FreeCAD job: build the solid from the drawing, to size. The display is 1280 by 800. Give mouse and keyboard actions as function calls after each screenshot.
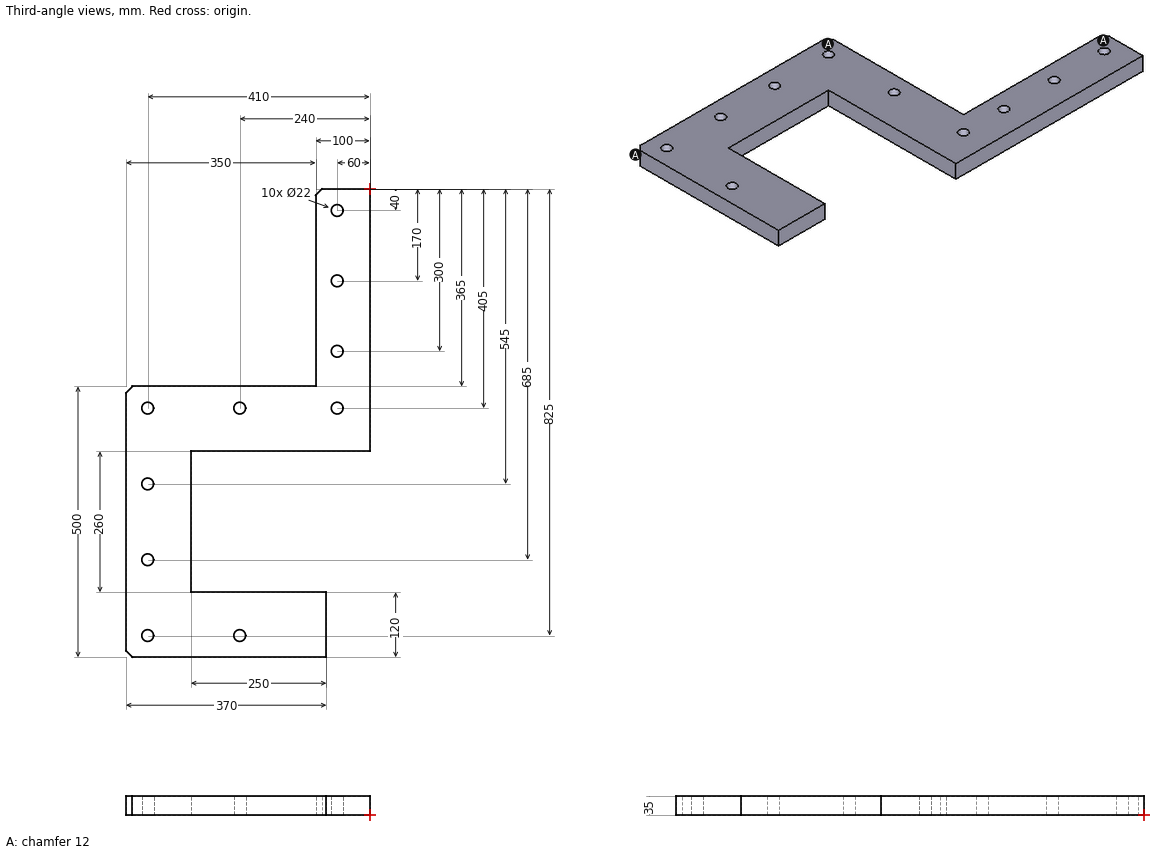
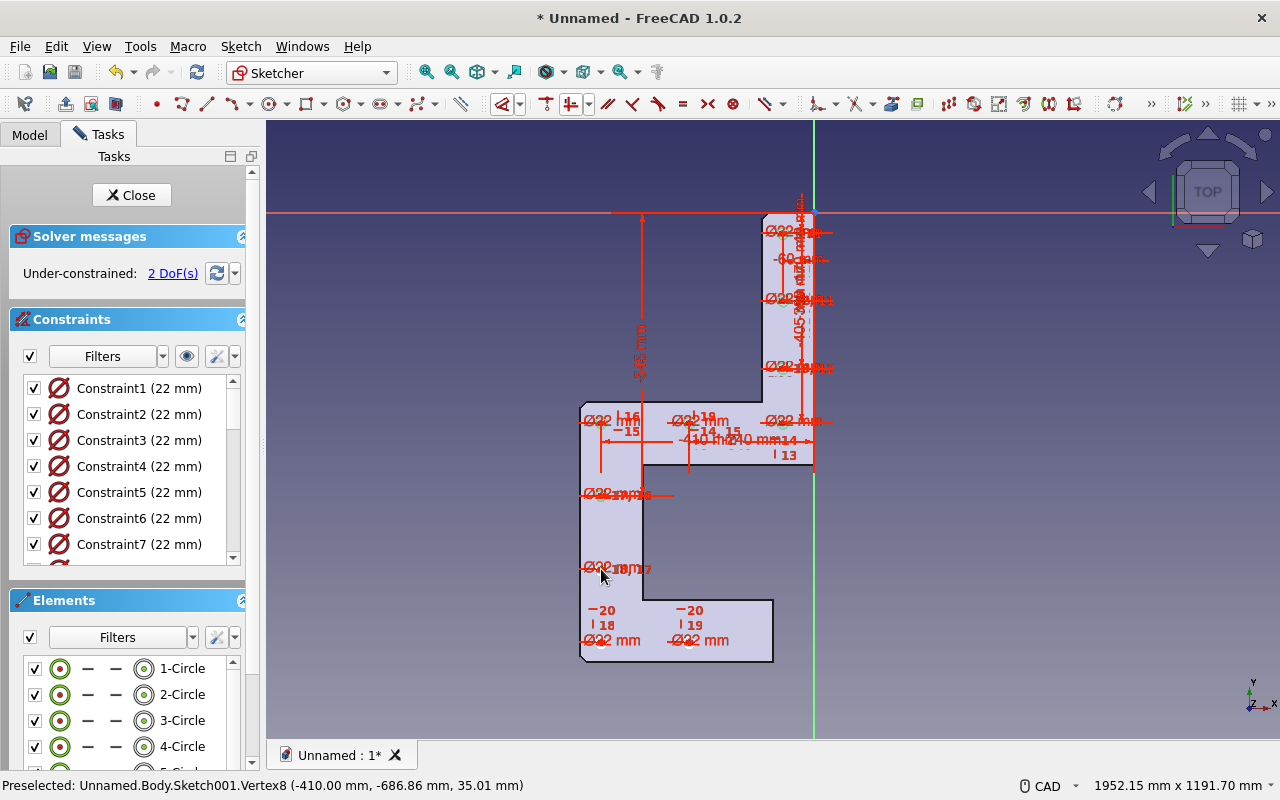
click(520, 104)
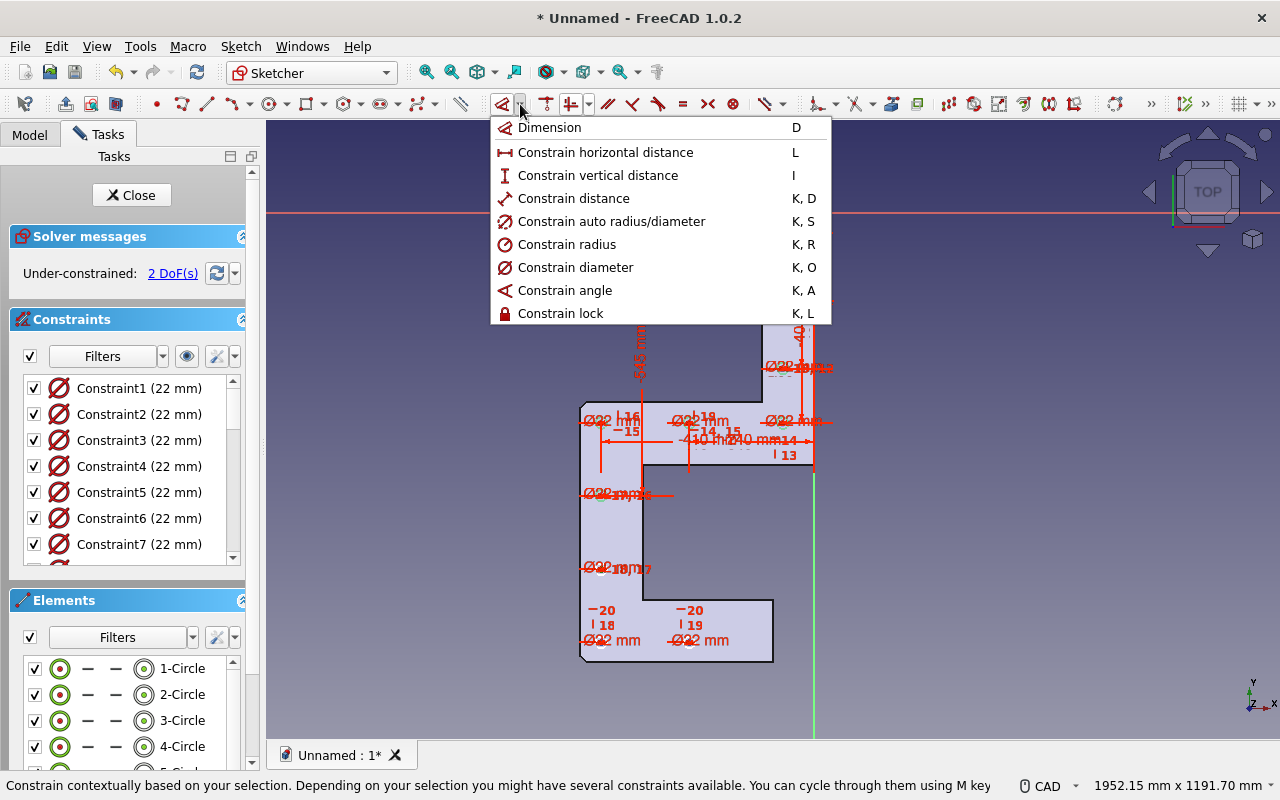
click(661, 176)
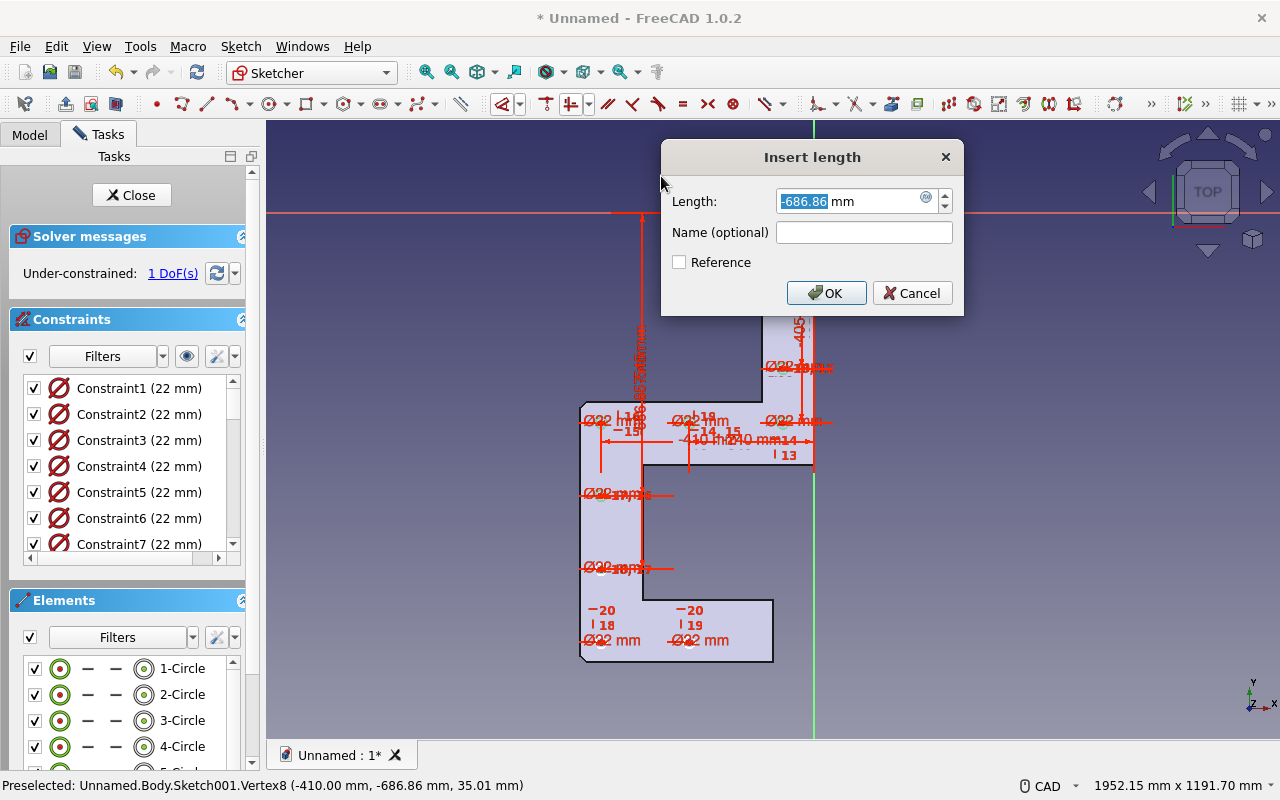
text(-685)
key(Return)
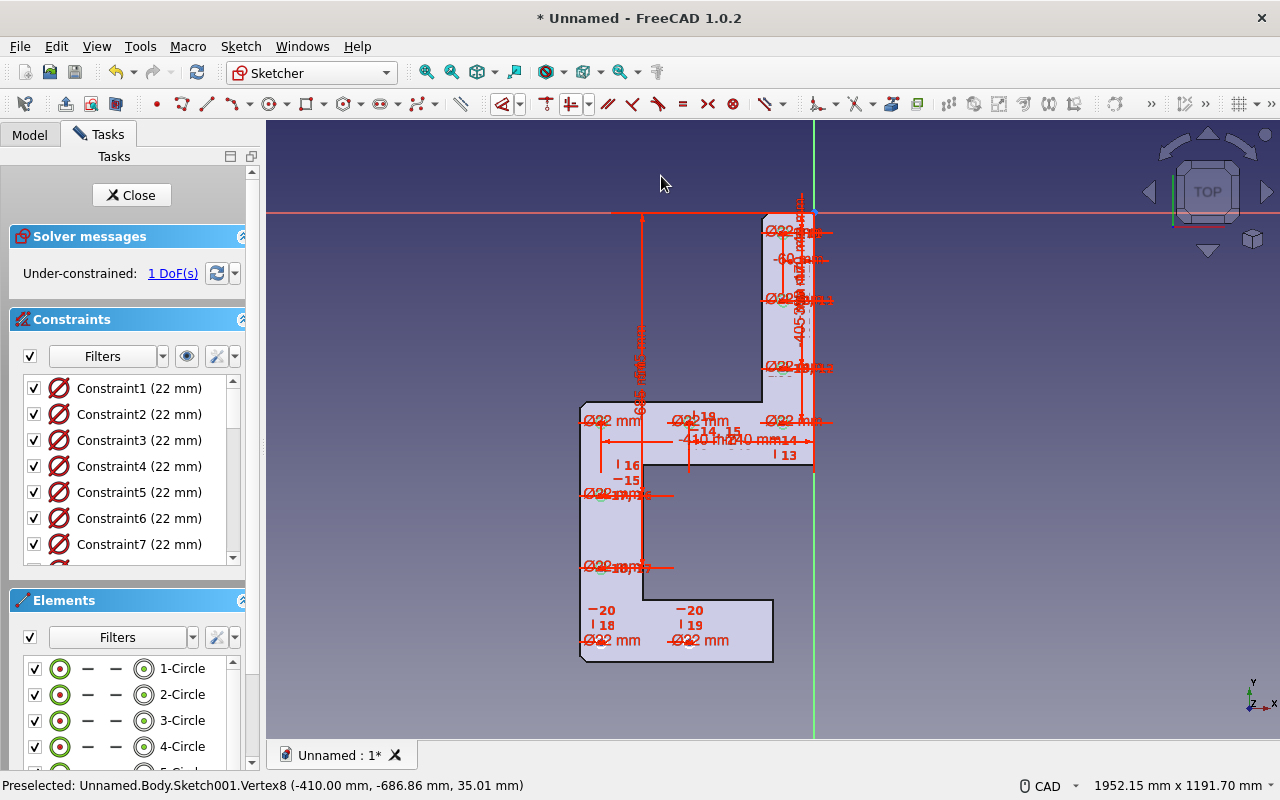
click(601, 642)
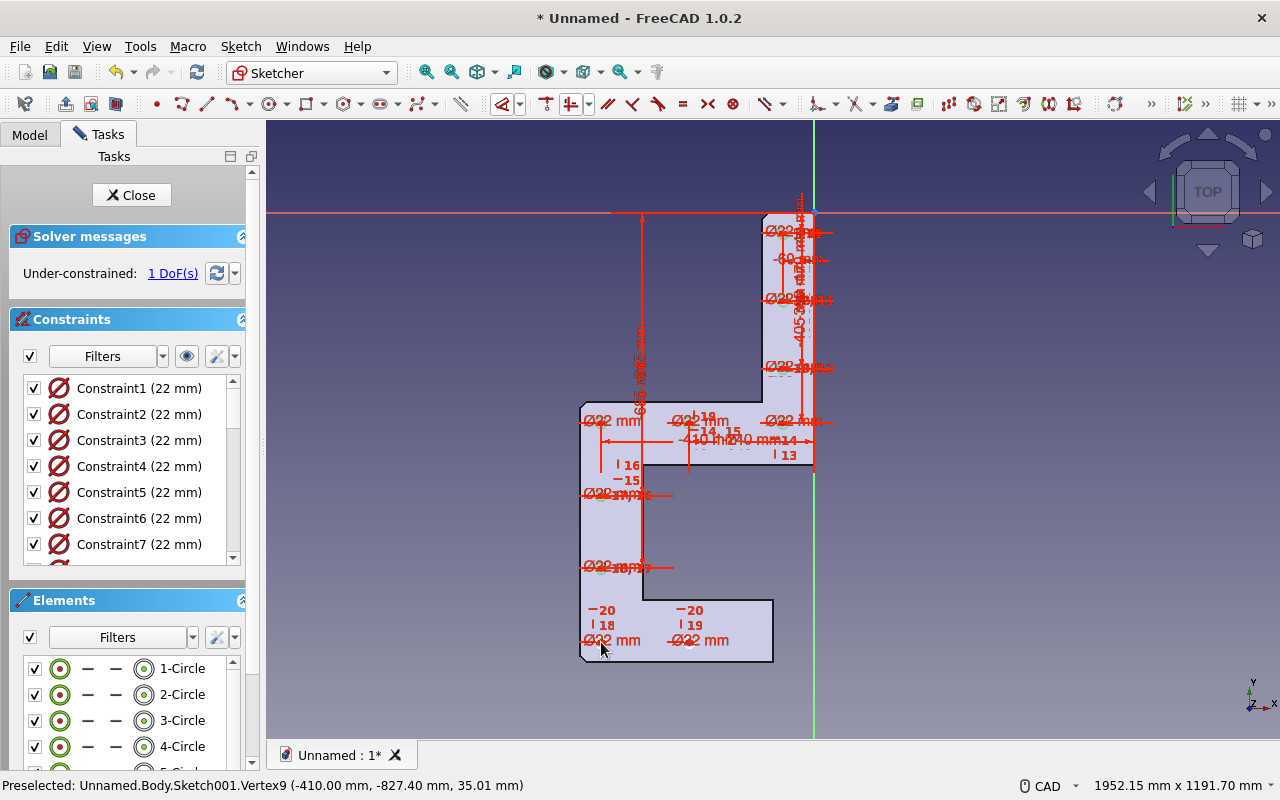
click(520, 104)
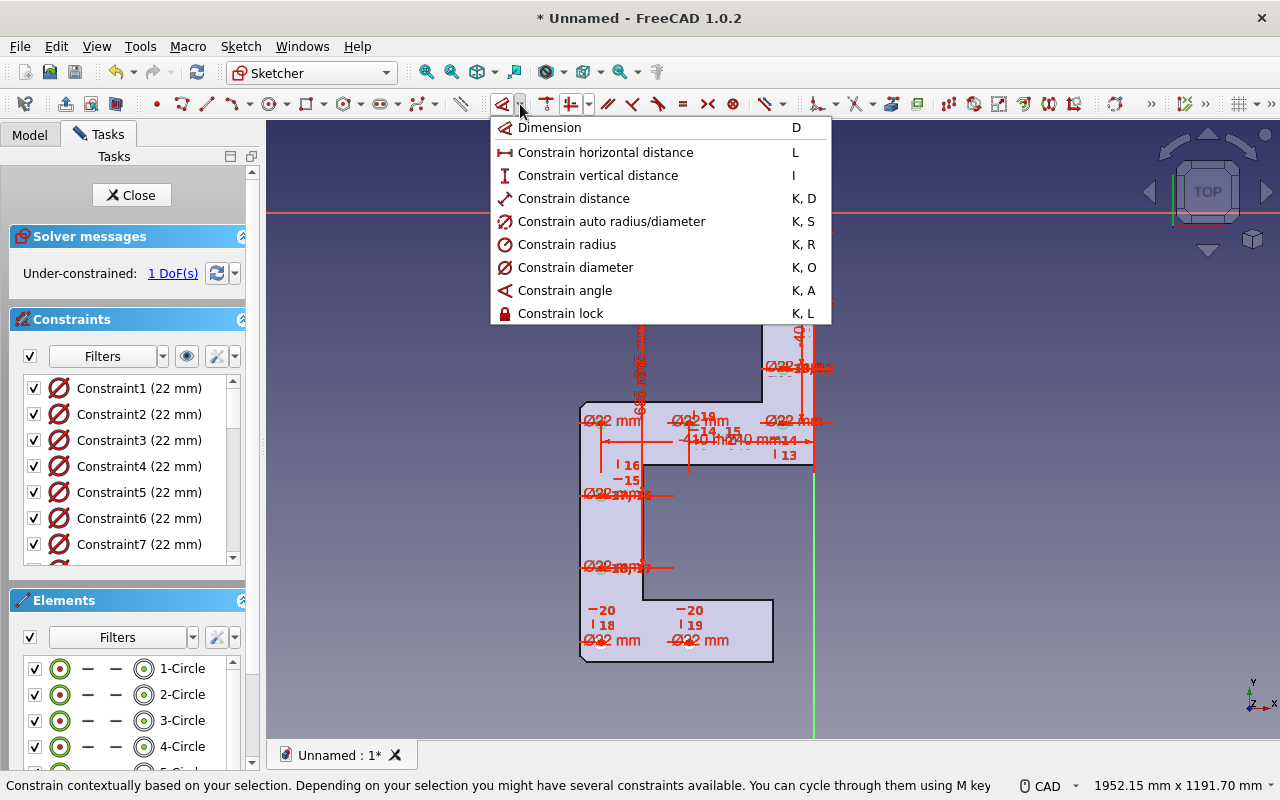
click(661, 176)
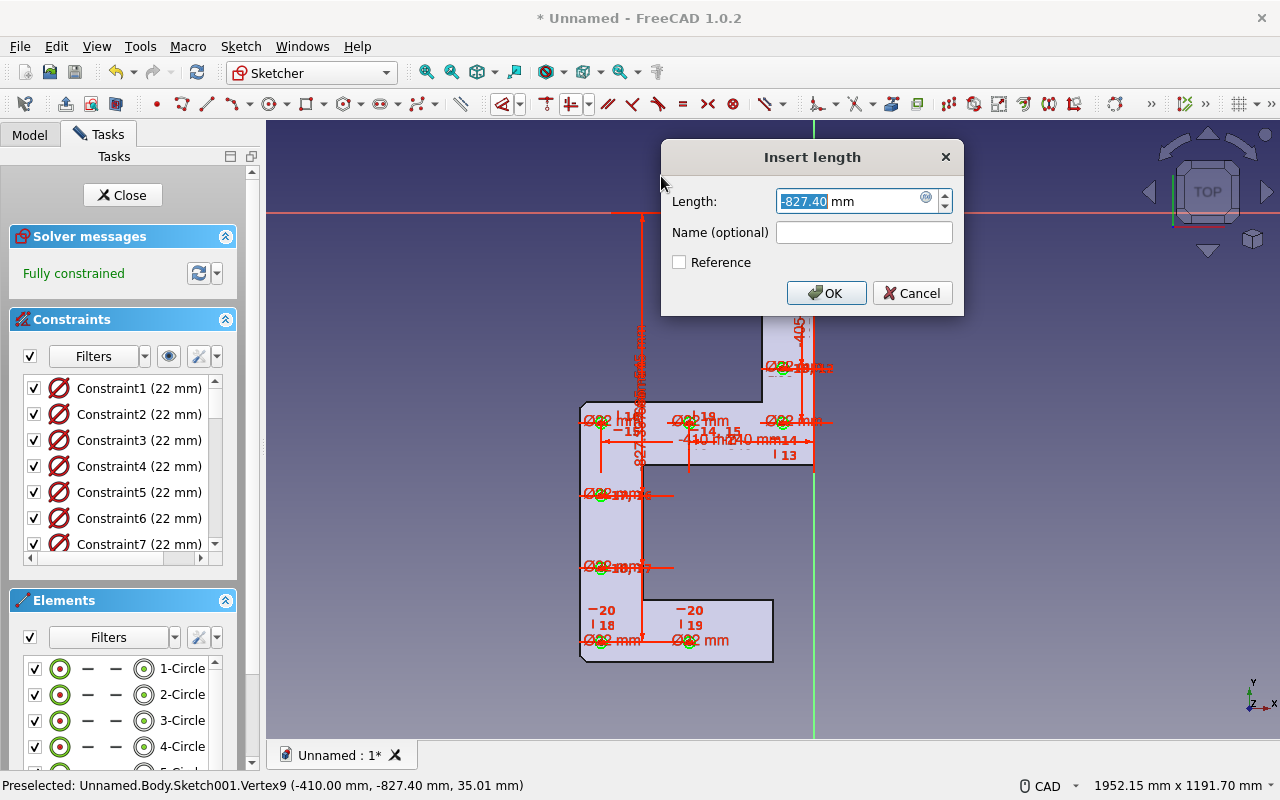
text(-825)
key(Return)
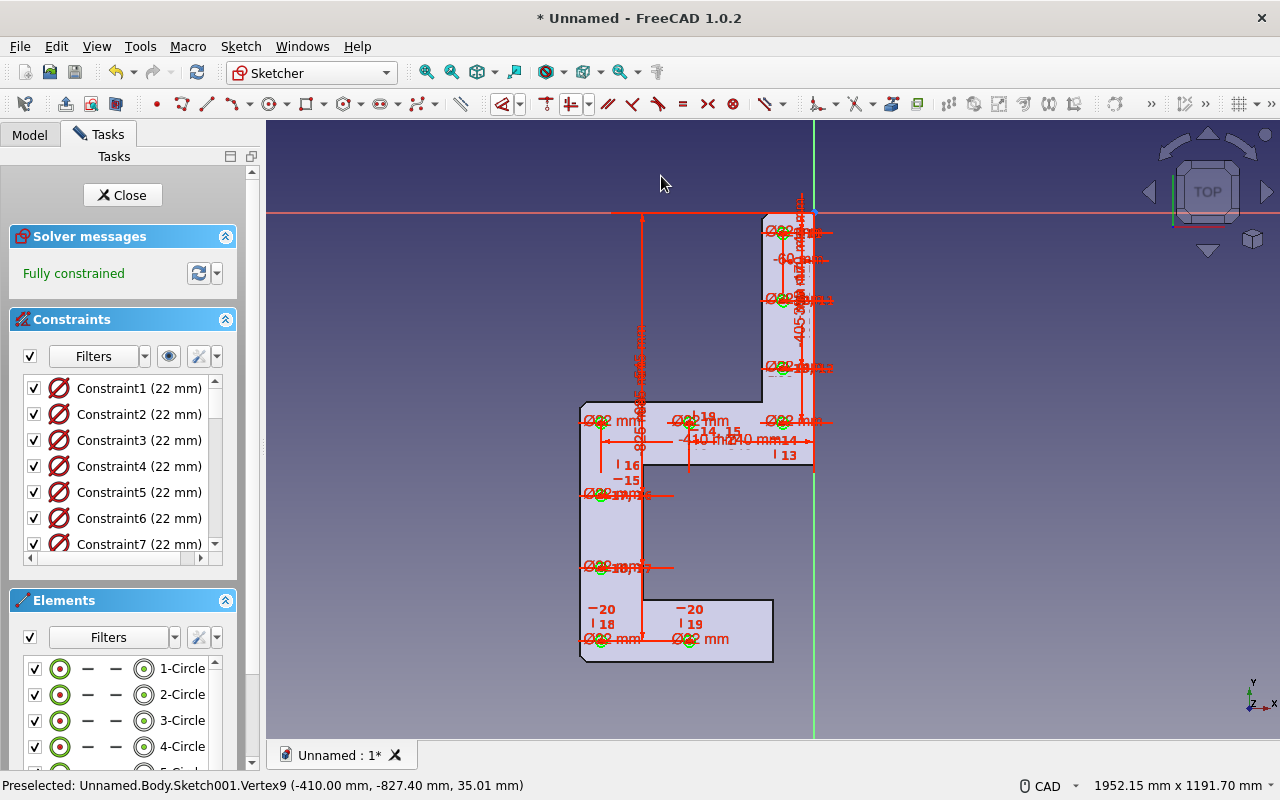
click(123, 195)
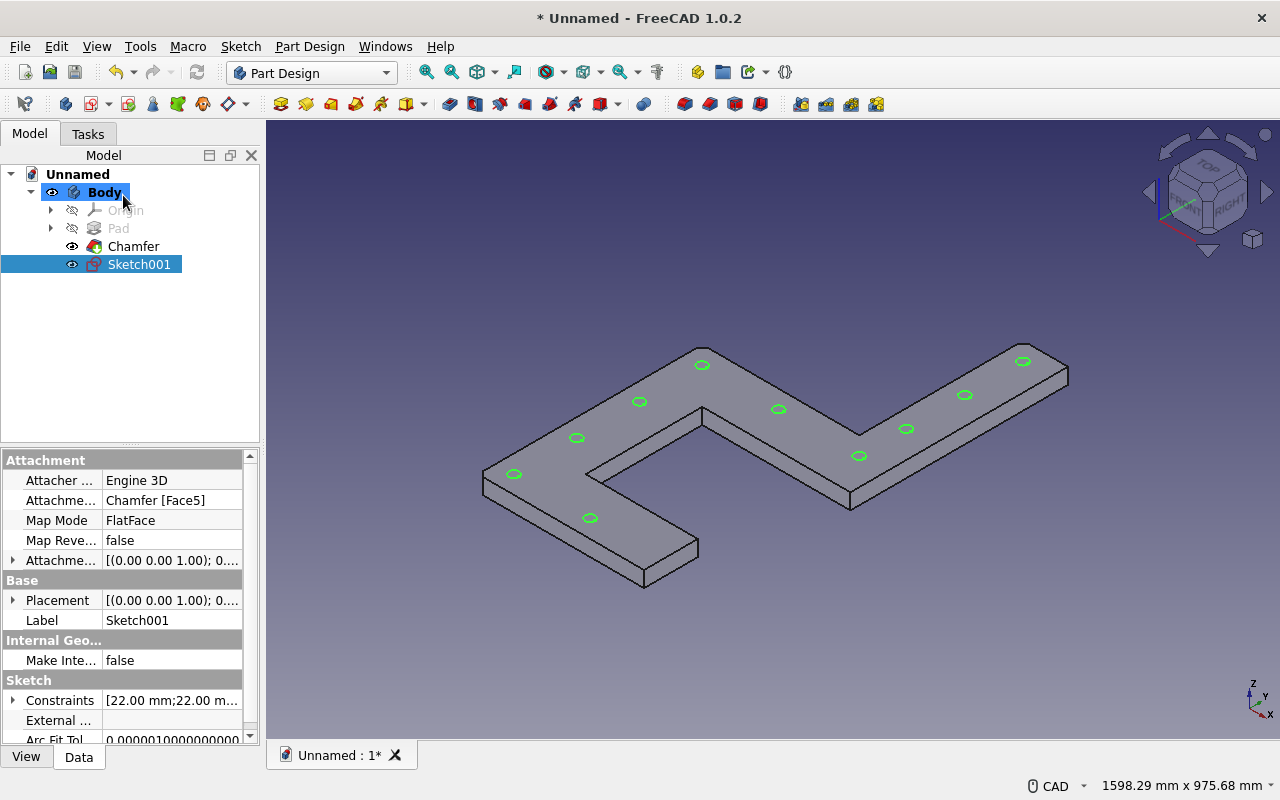
click(450, 104)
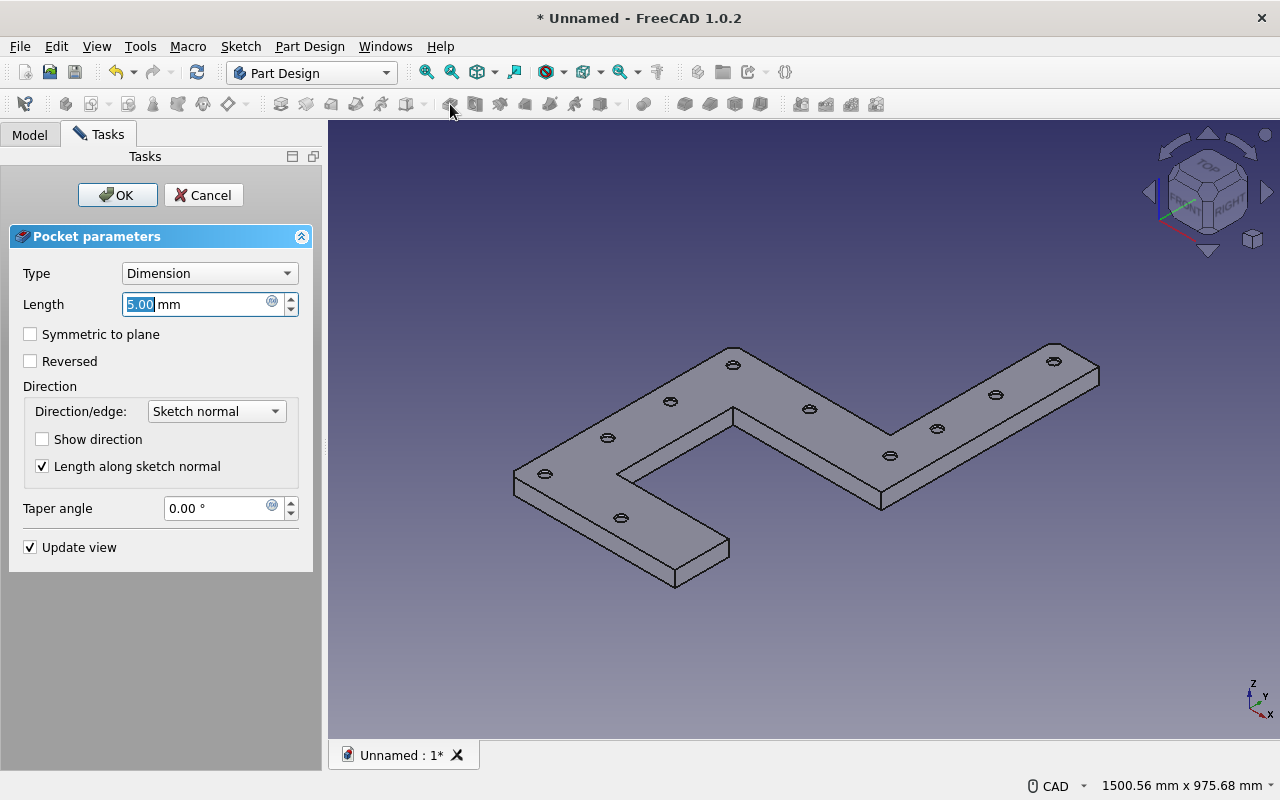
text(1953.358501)
key(Tab)